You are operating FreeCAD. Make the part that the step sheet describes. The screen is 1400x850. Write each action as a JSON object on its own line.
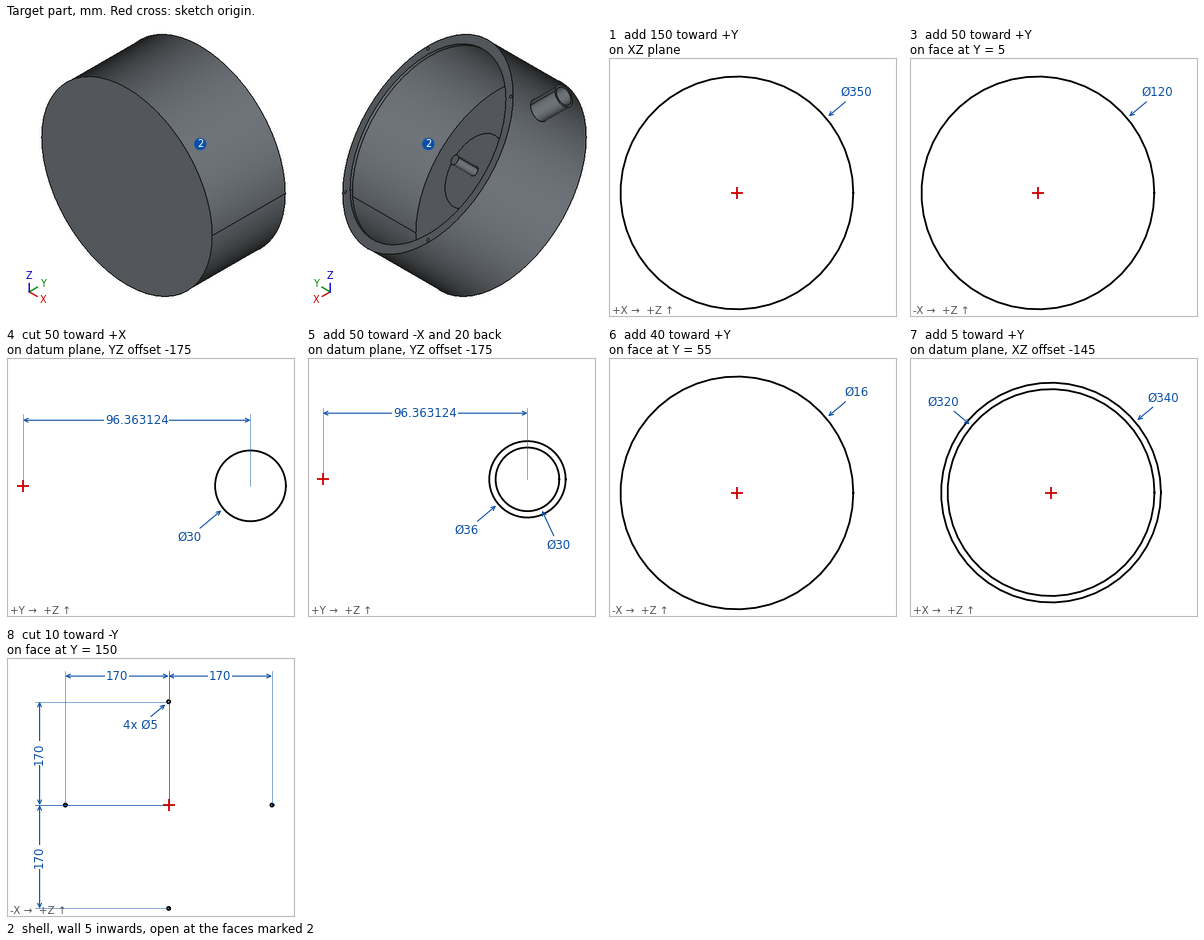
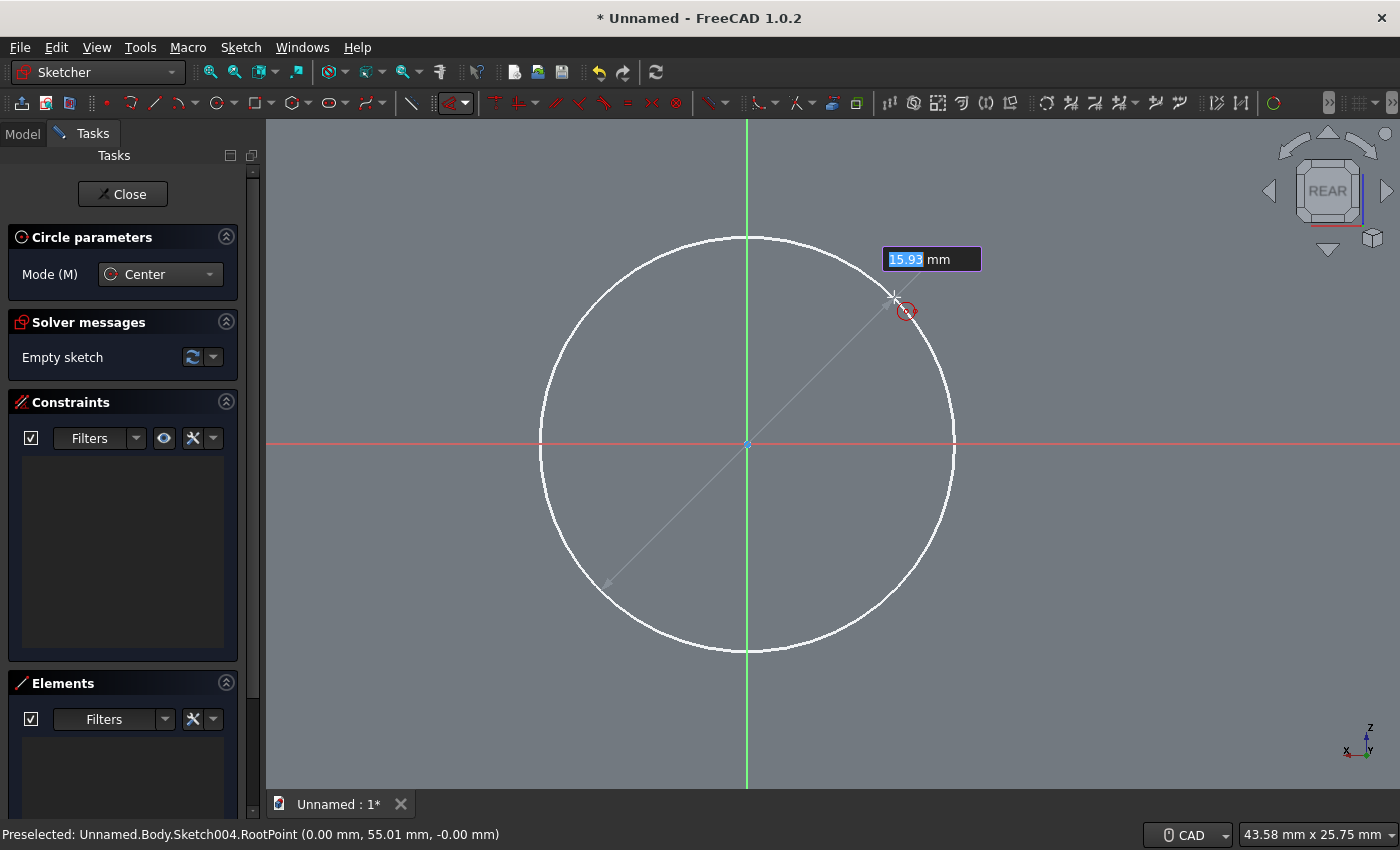
{"action": "type", "text": "16"}
{"action": "key", "text": "Return"}
{"action": "key", "text": "Escape"}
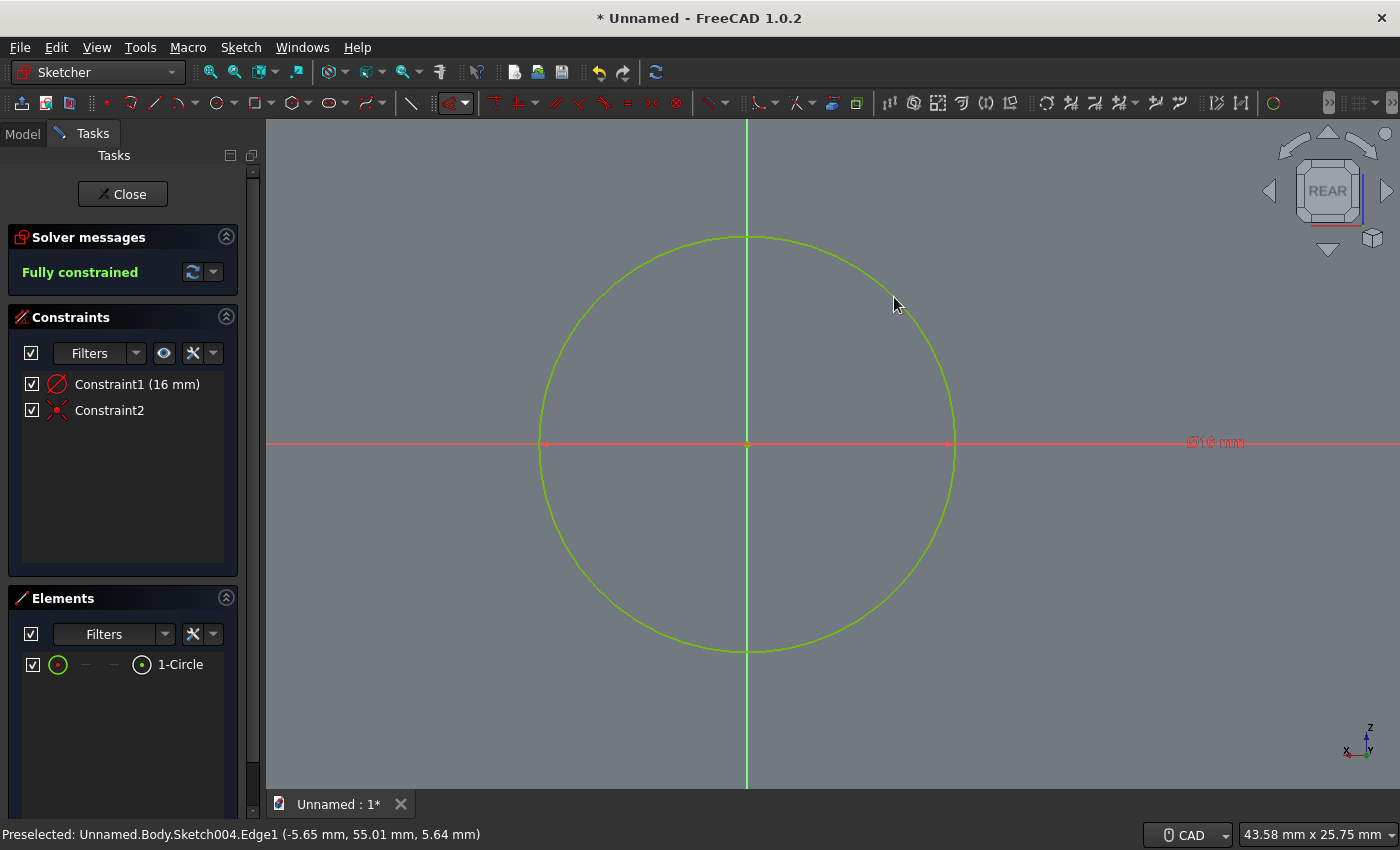
{"action": "left_click", "coordinate": [123, 194]}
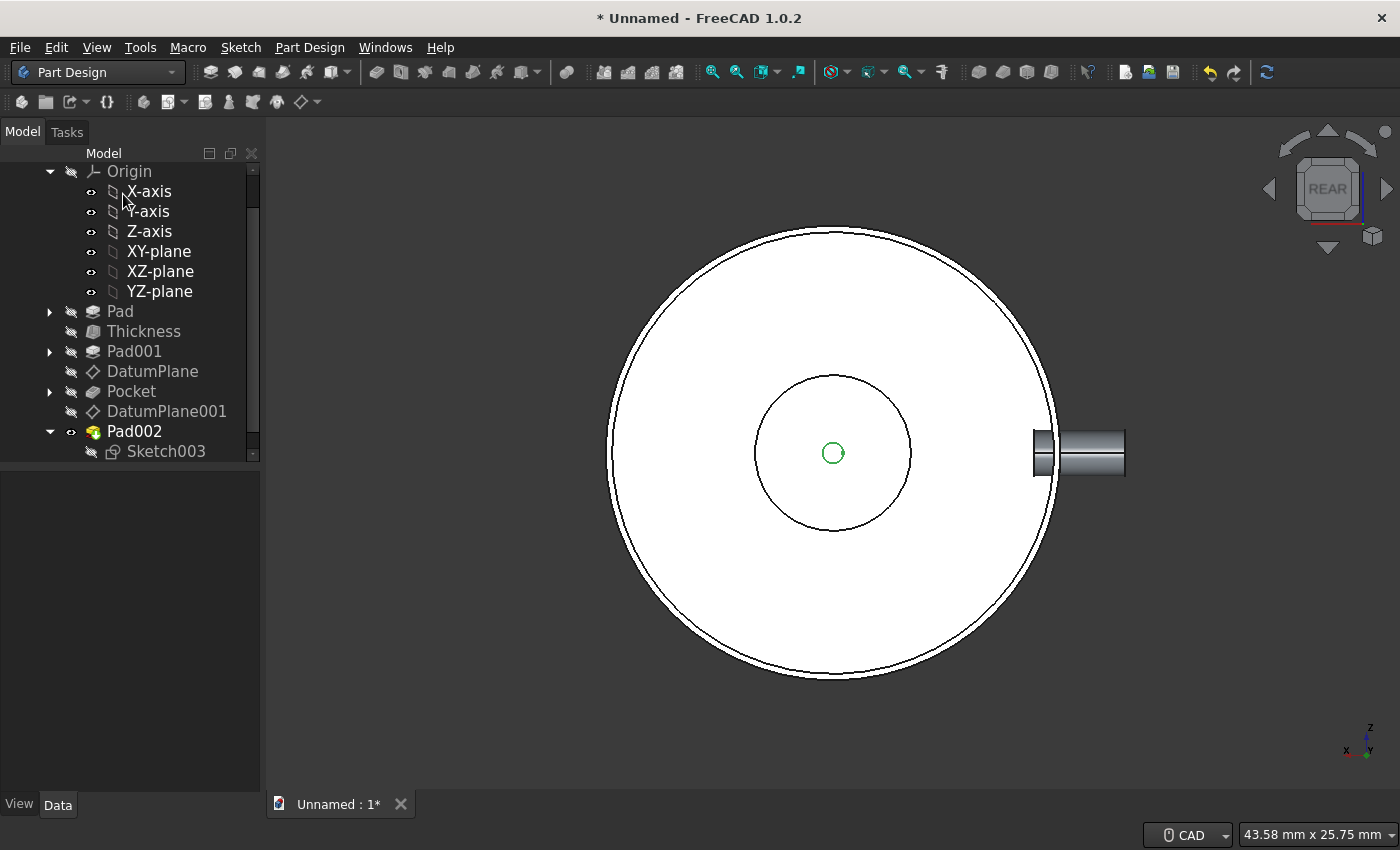
{"action": "left_click", "coordinate": [212, 72]}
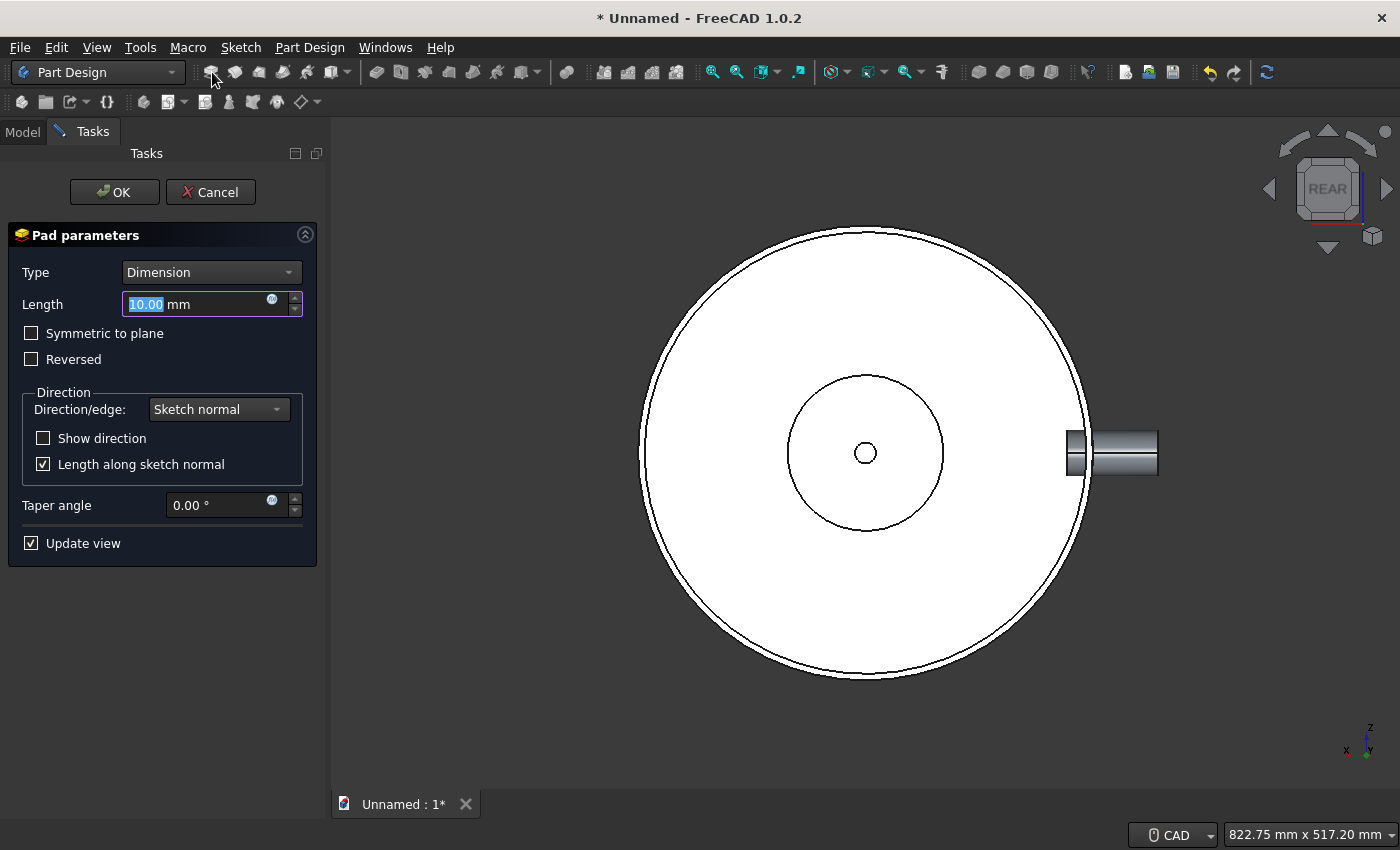
{"action": "type", "text": "40"}
{"action": "key", "text": "Tab"}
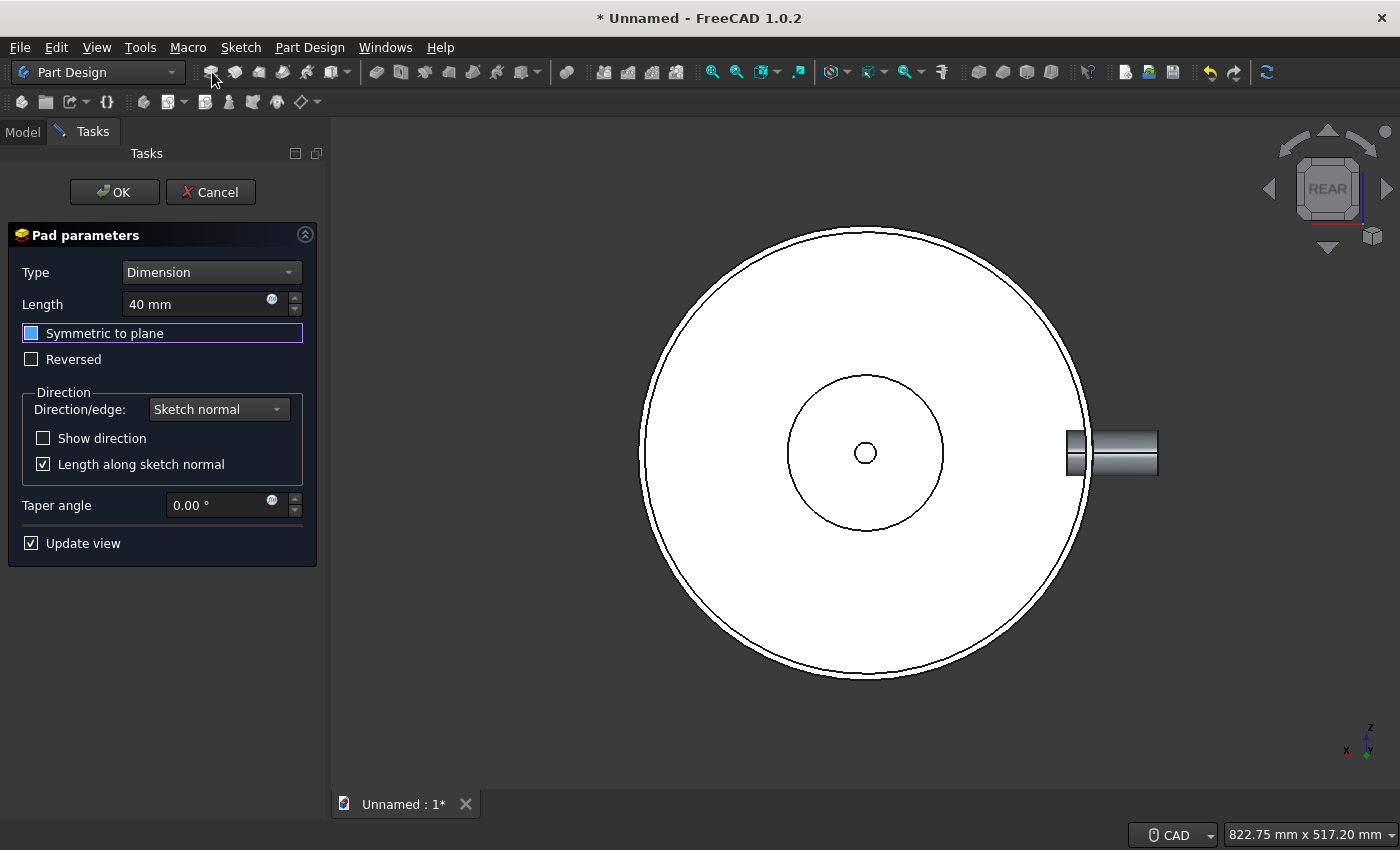
{"action": "left_click", "coordinate": [115, 192]}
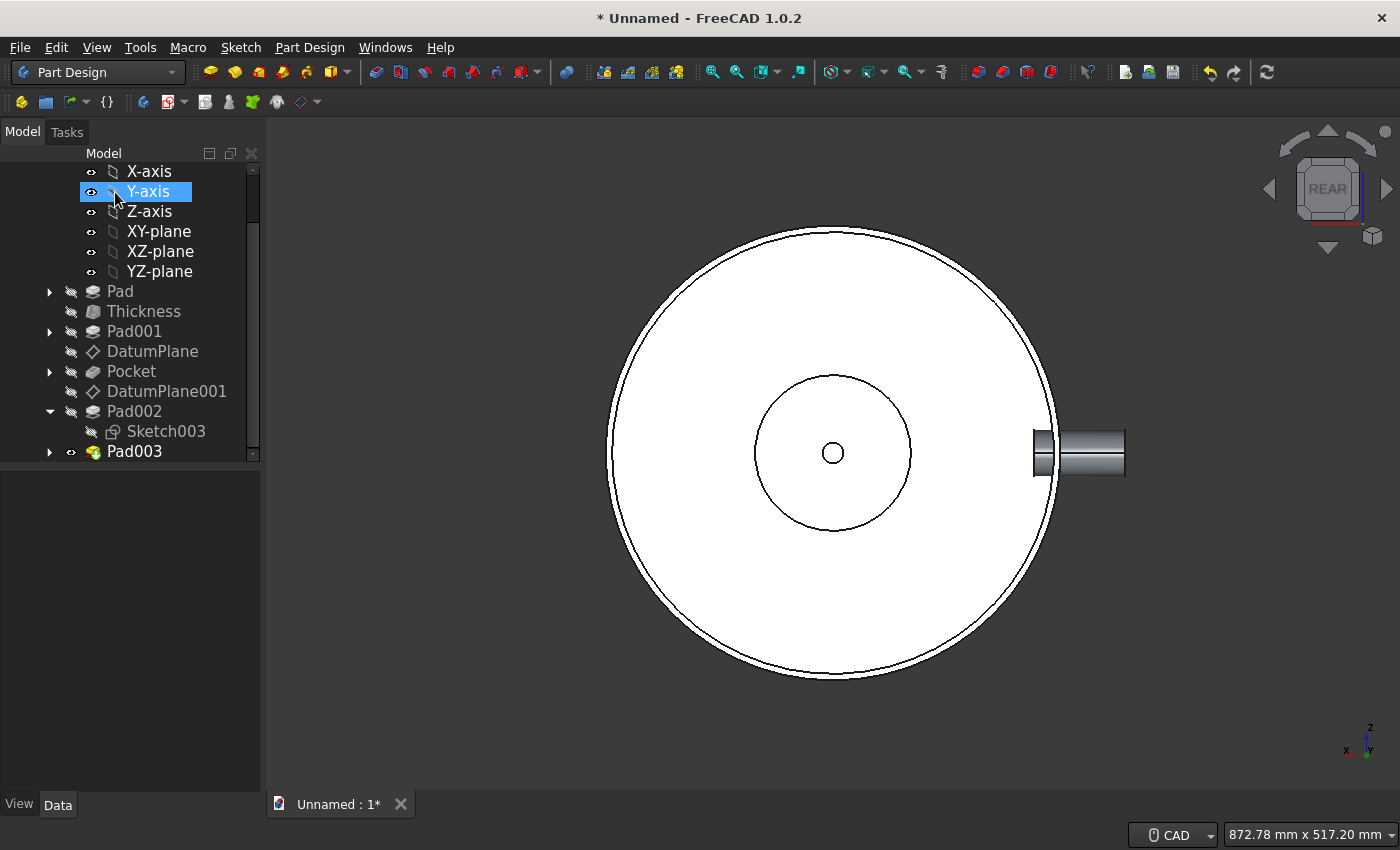
{"action": "scroll", "coordinate": [160, 307], "scroll_direction": "down", "scroll_amount": 3}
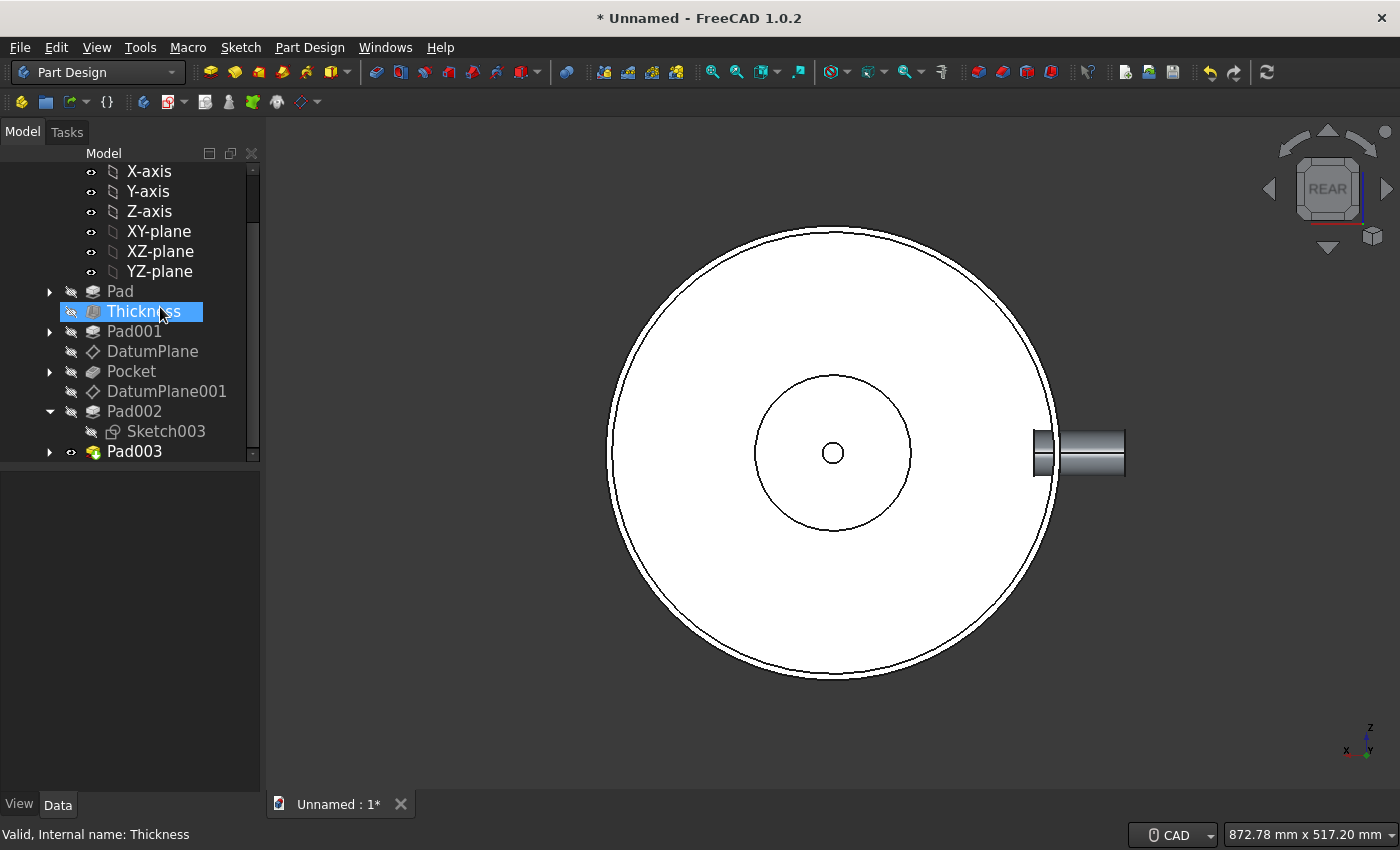
{"action": "scroll", "coordinate": [160, 307], "scroll_direction": "up", "scroll_amount": 15}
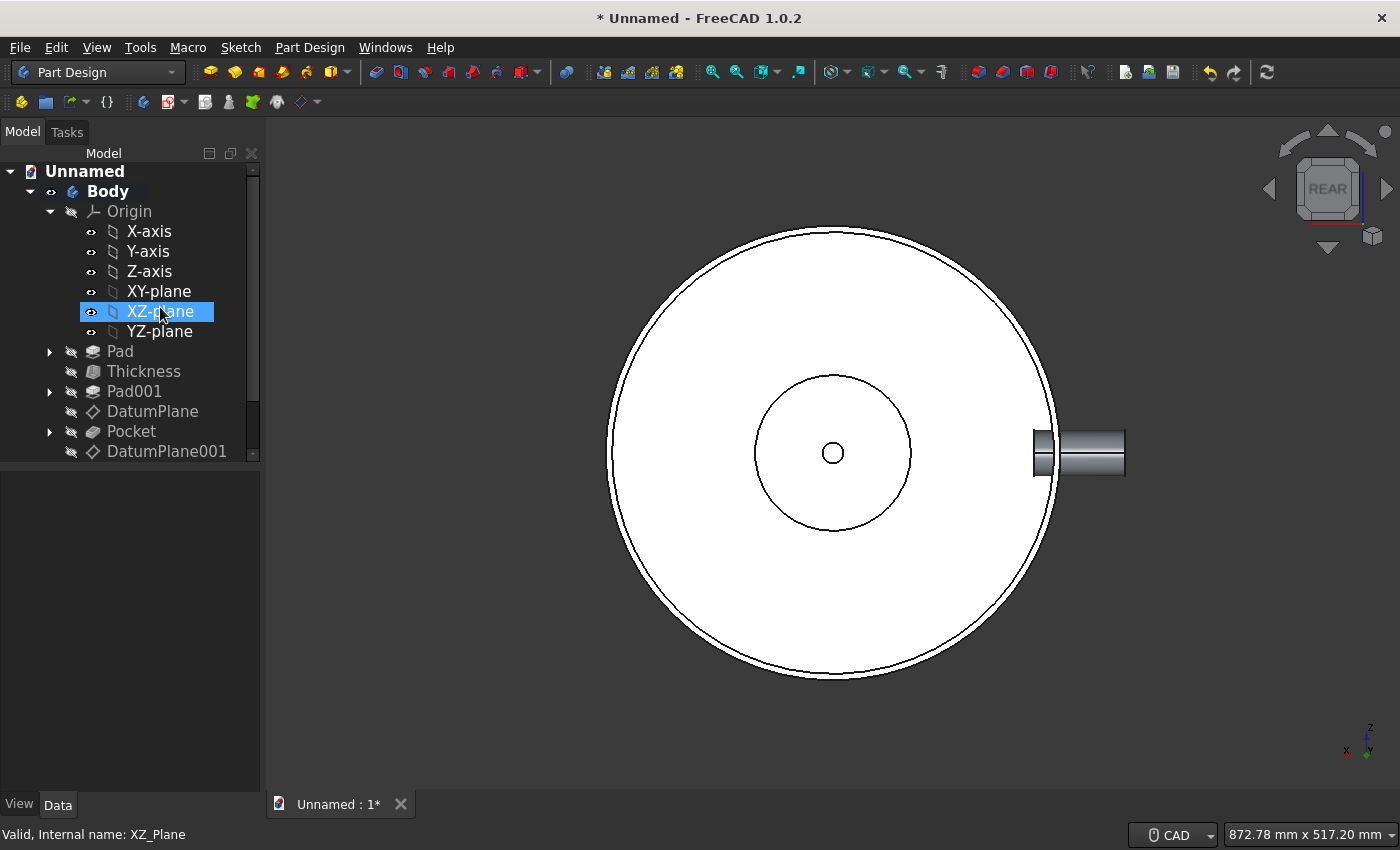
{"action": "left_click", "coordinate": [136, 312]}